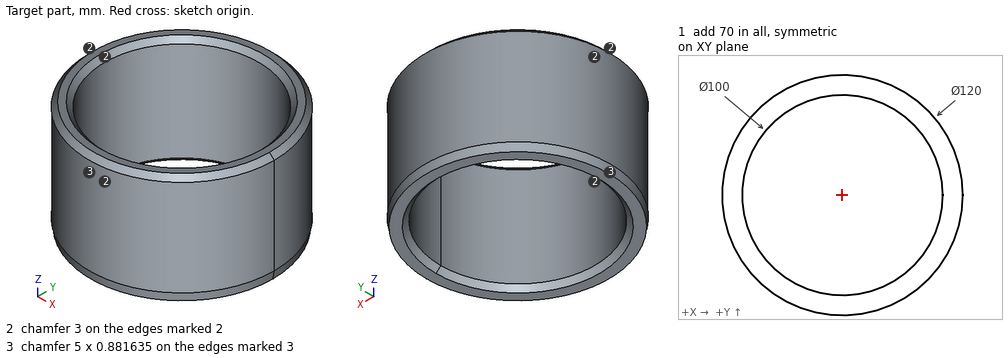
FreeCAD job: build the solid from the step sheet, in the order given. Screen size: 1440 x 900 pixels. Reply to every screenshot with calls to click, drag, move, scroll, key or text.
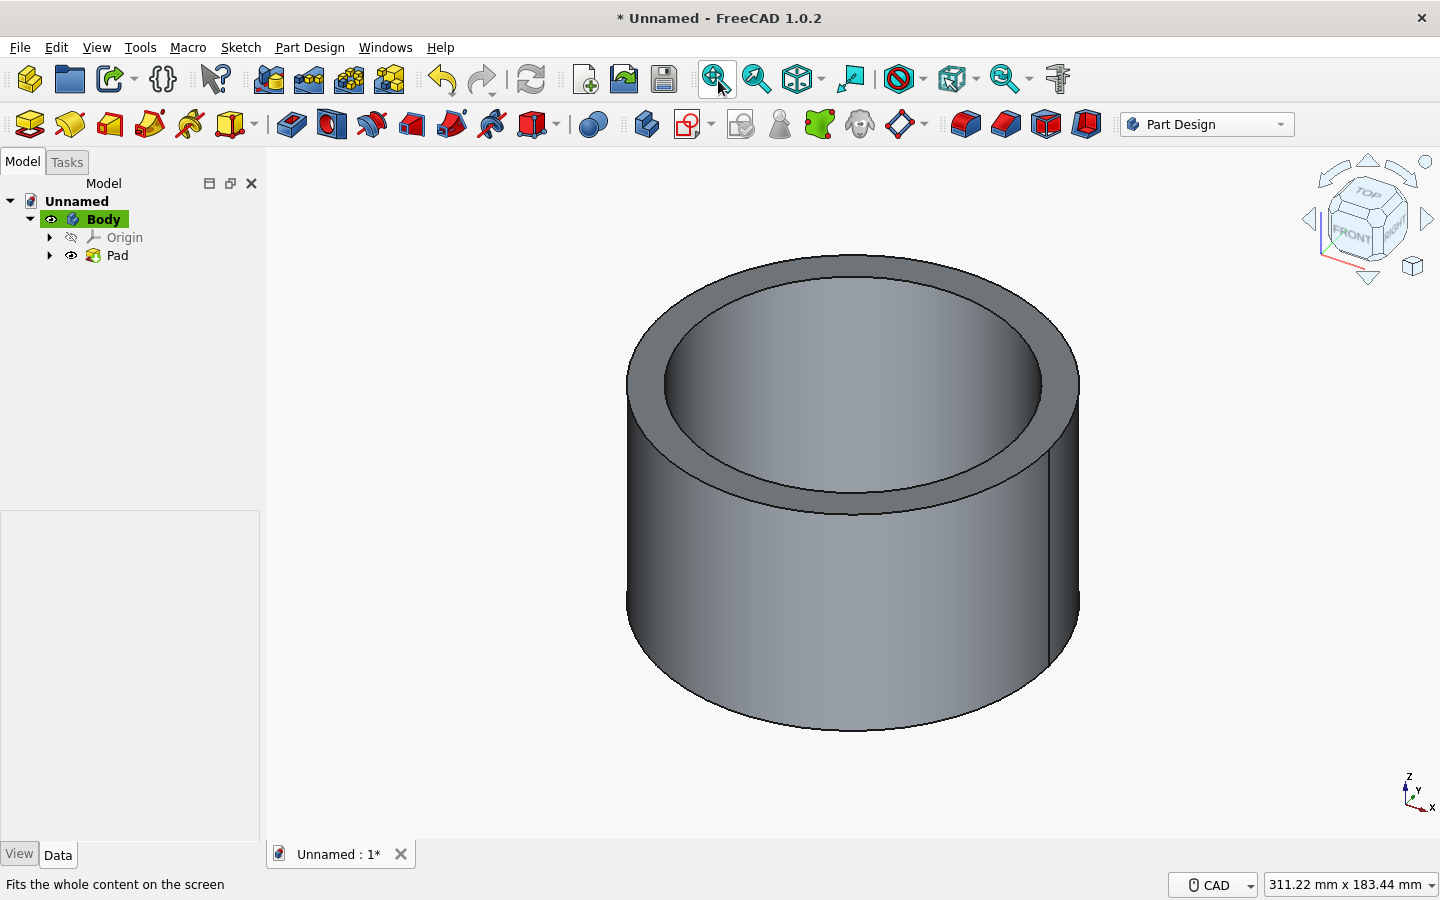
click(628, 397)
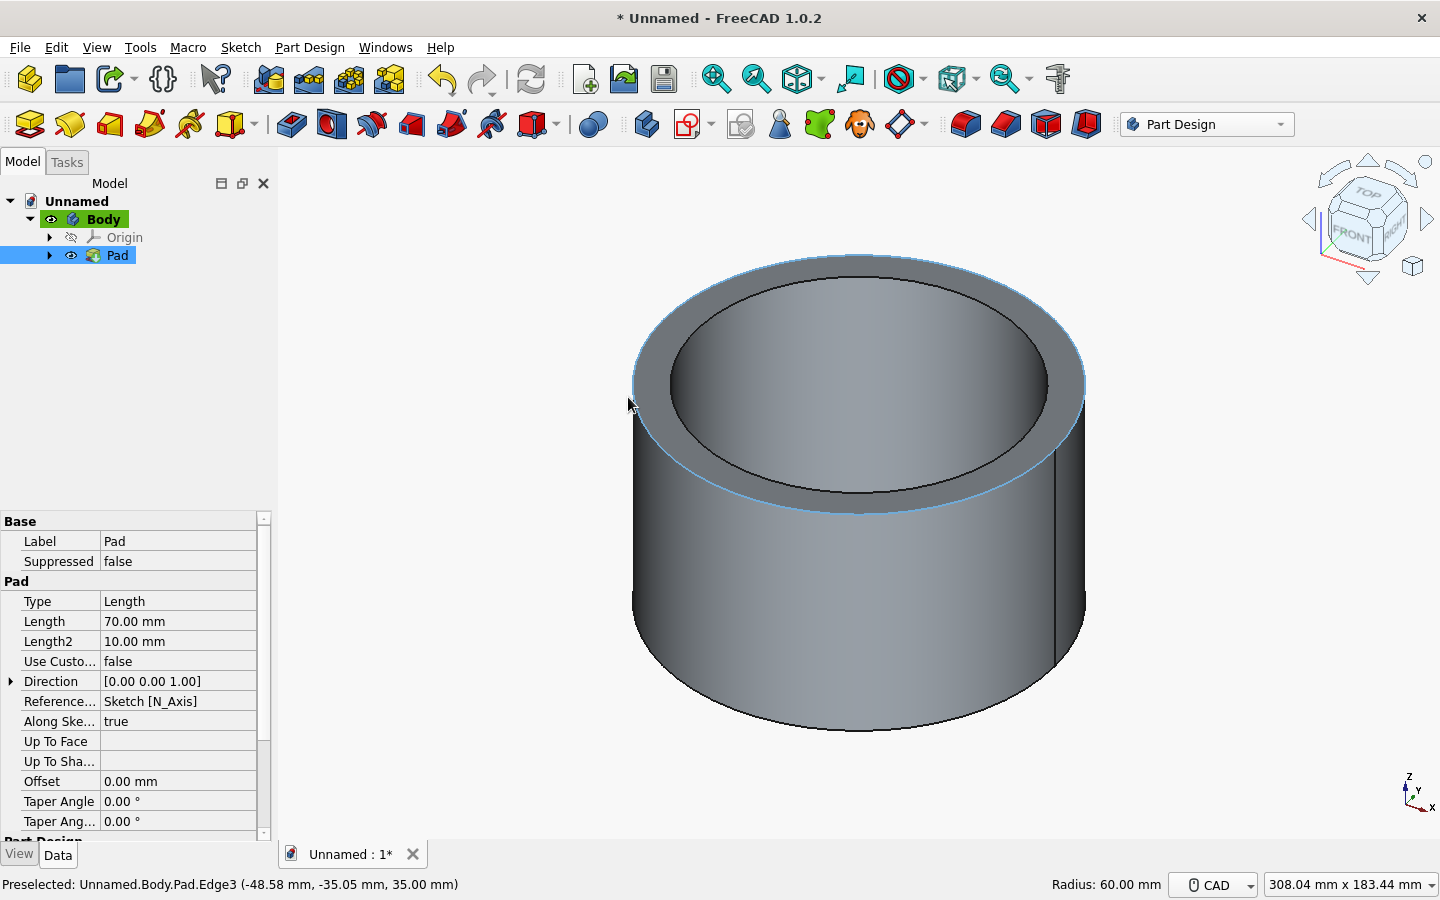
click(696, 330, ctrl)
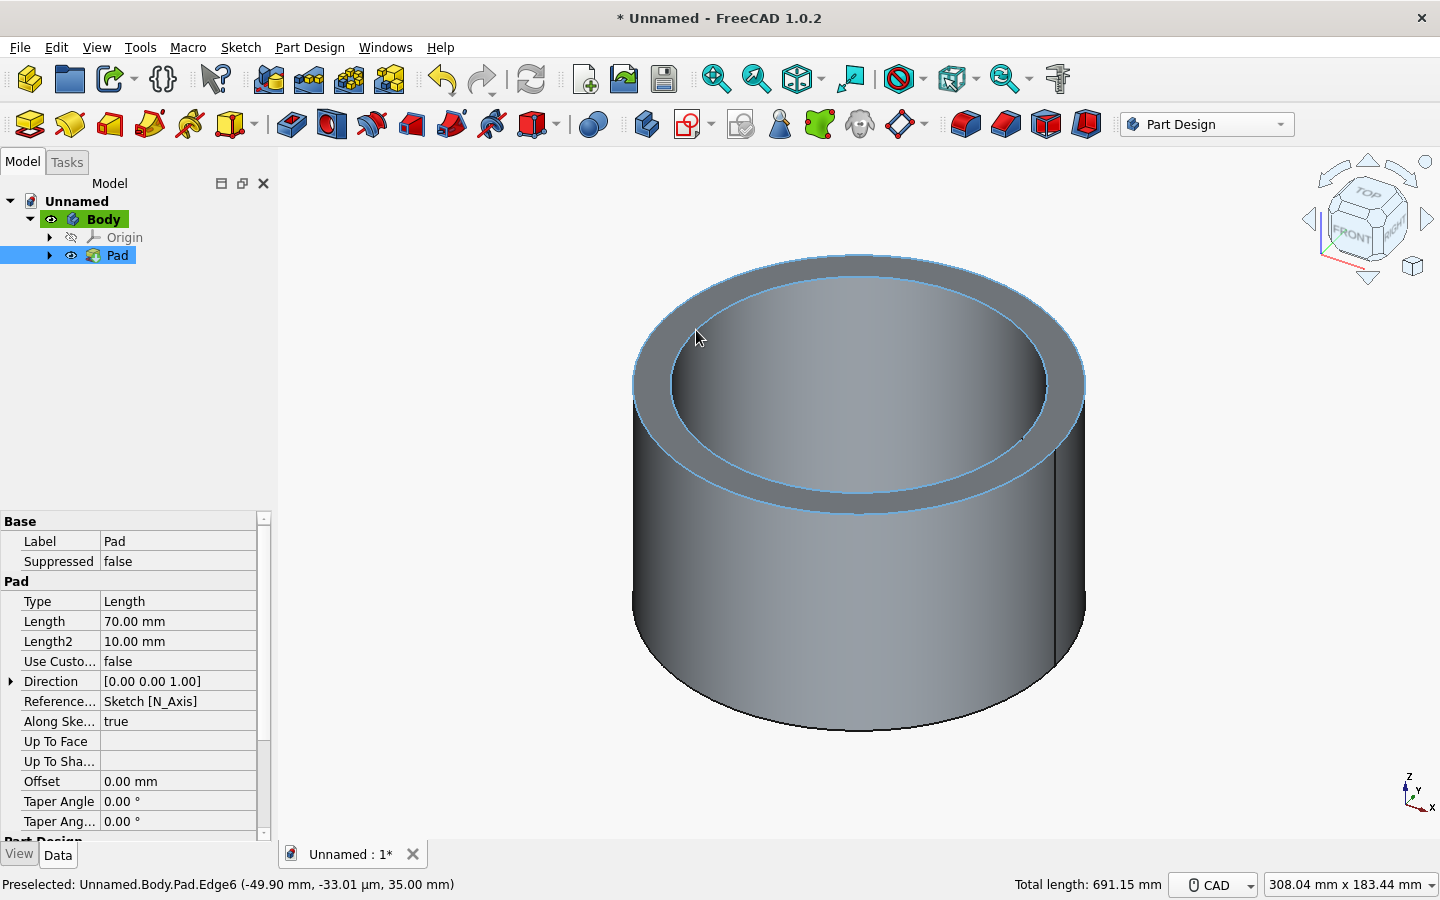
key(0)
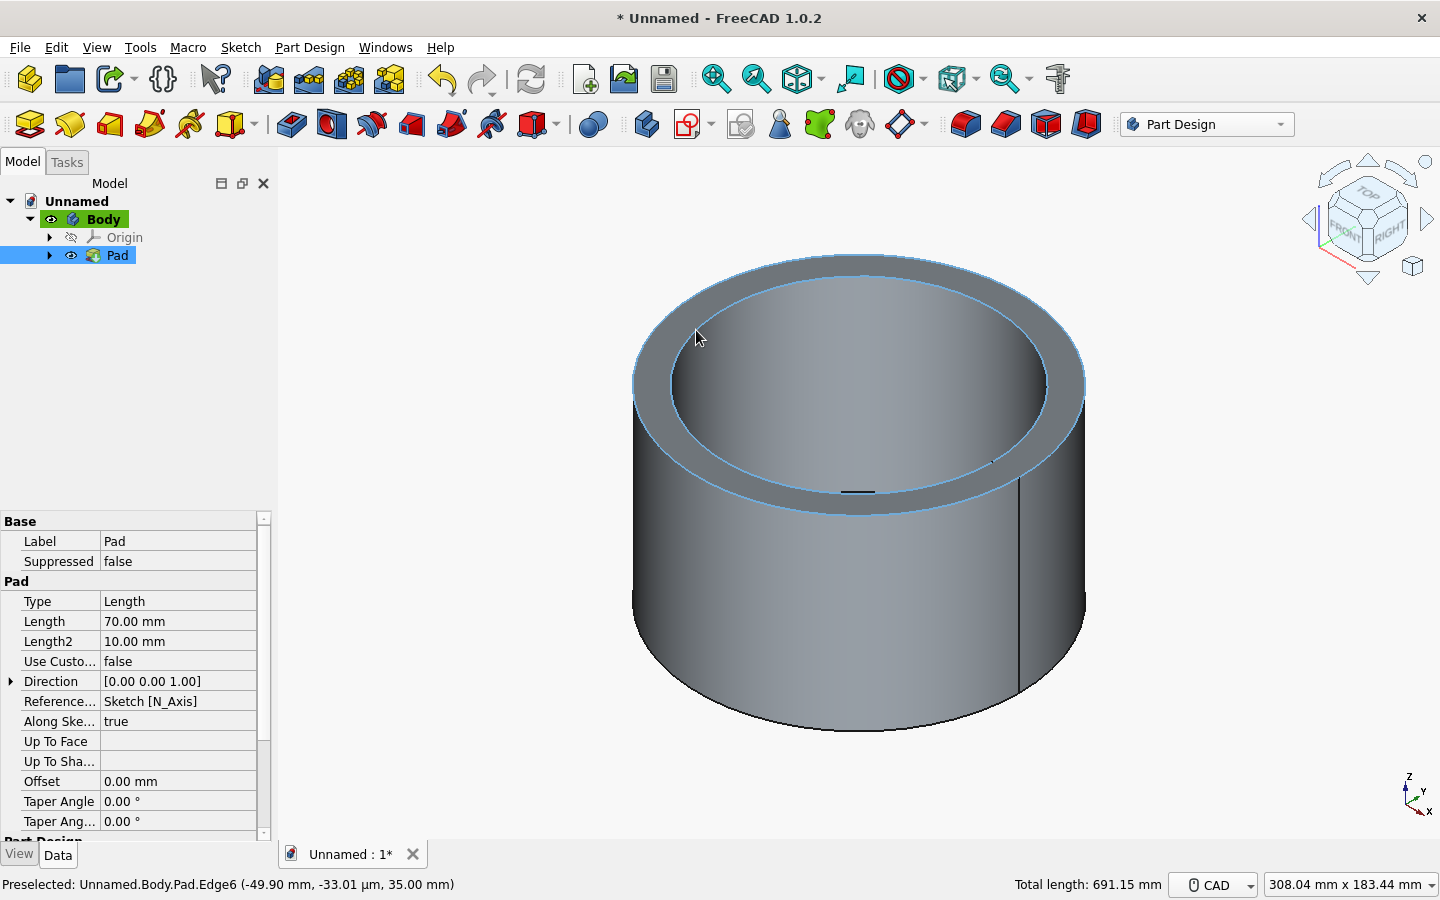
key(2)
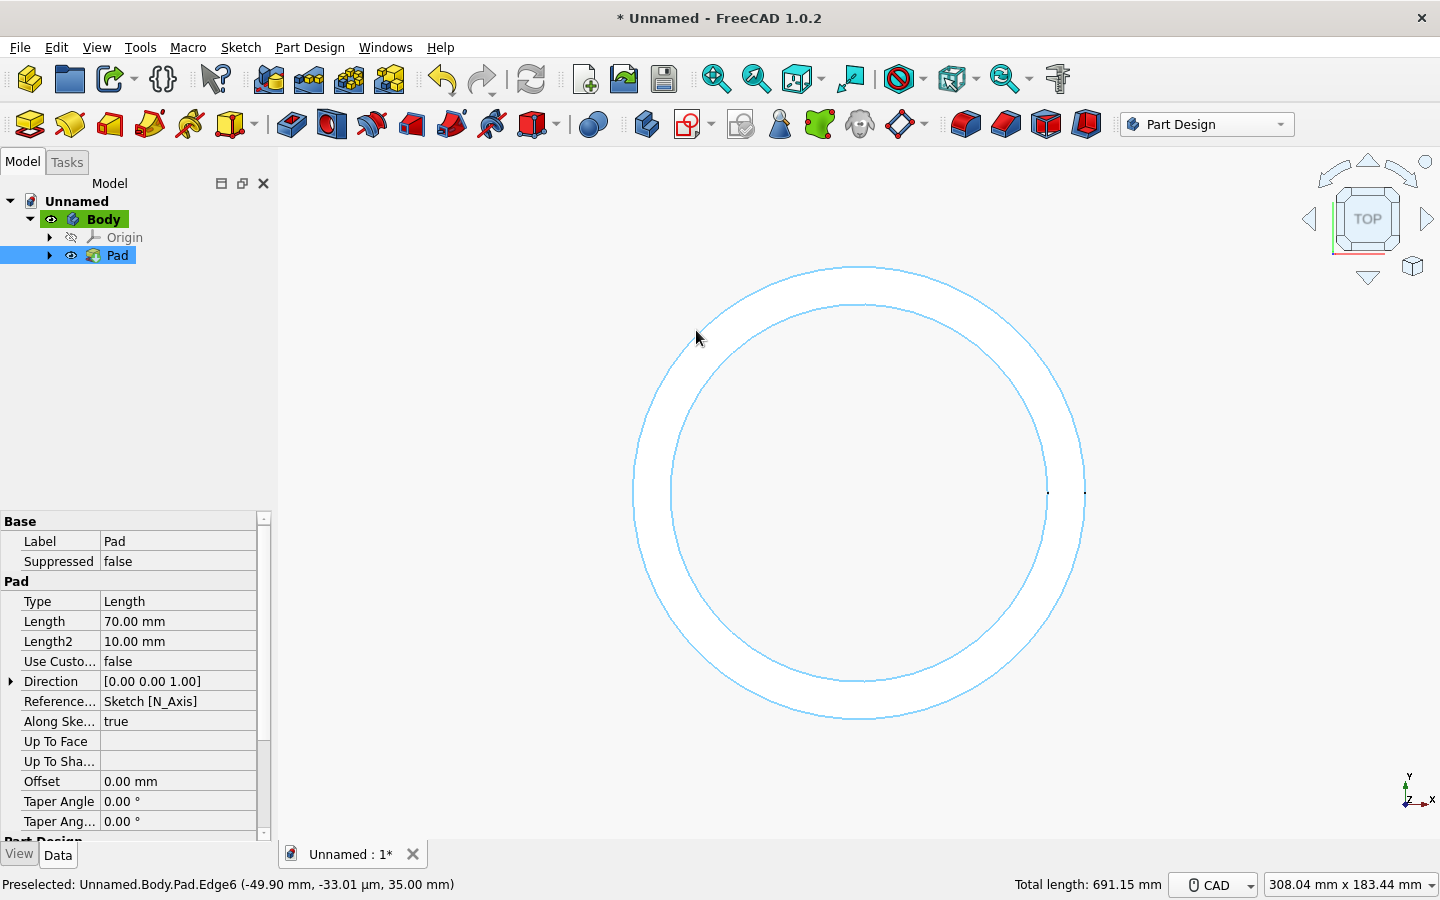
key(1)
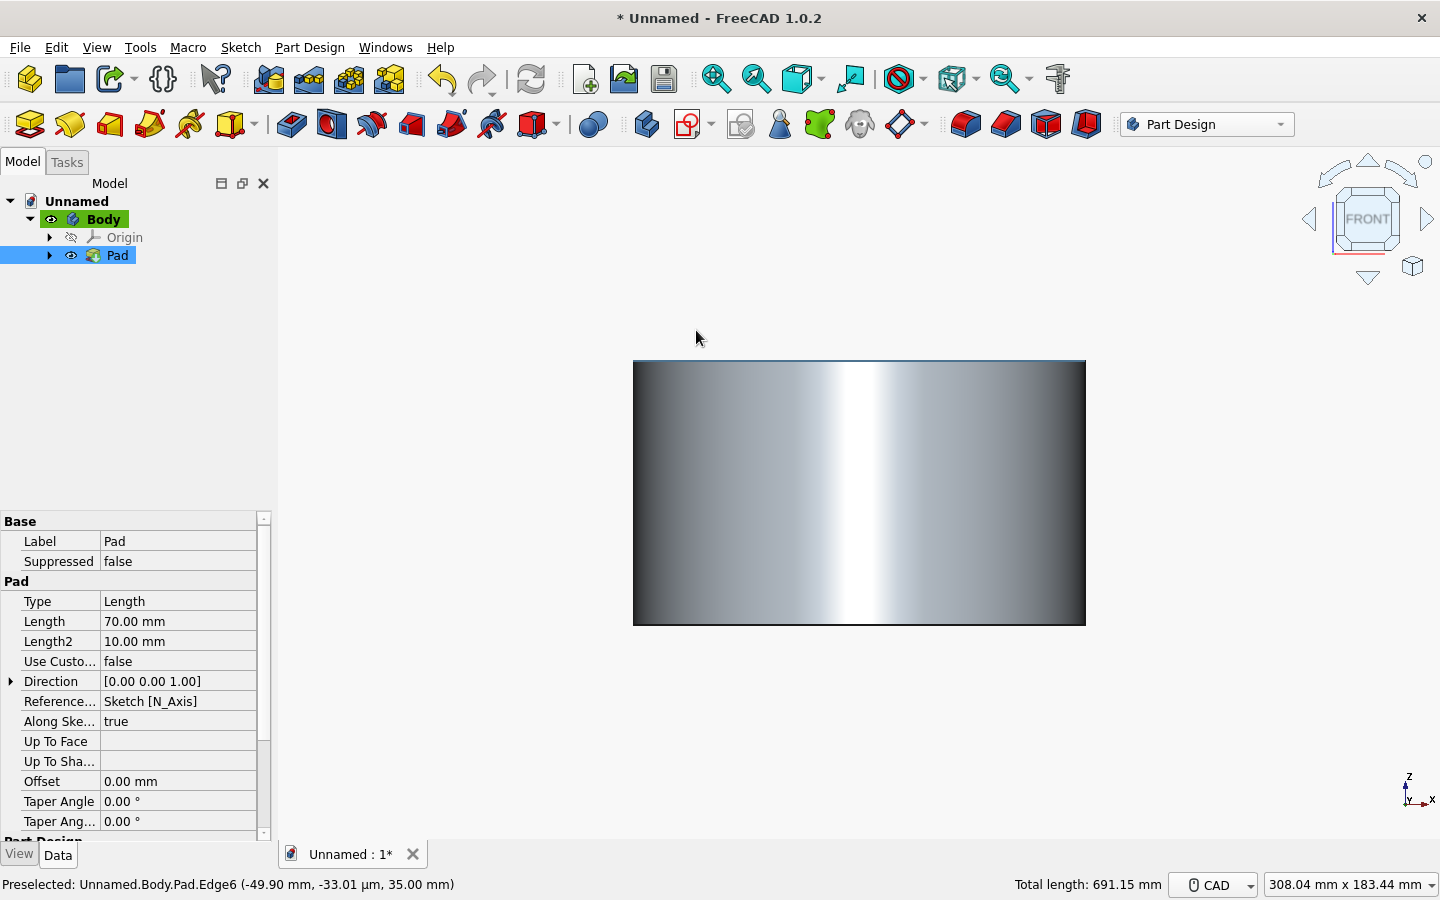
click(718, 80)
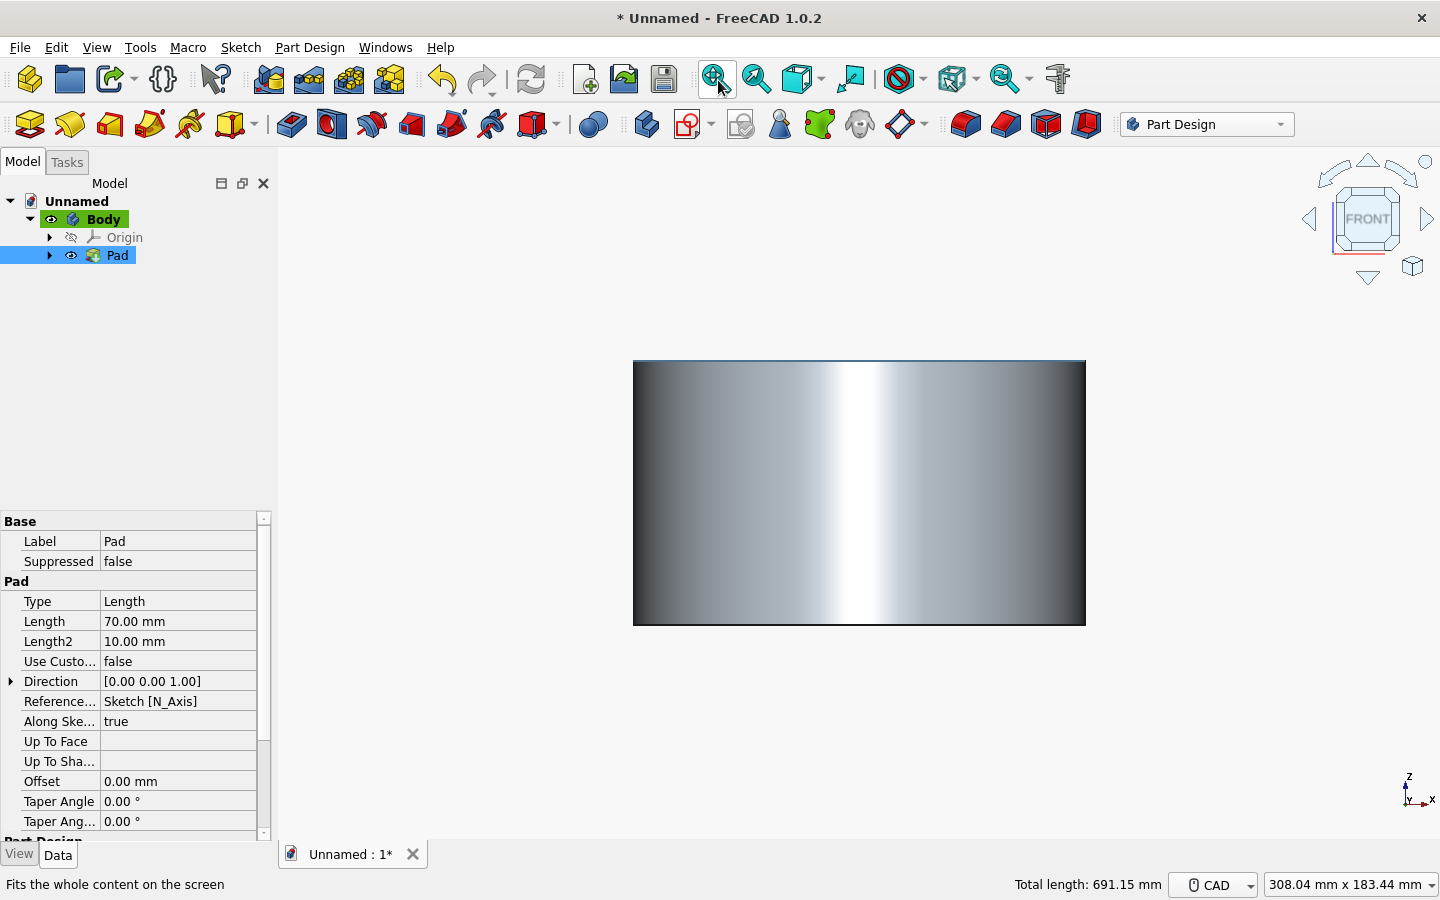
key(3)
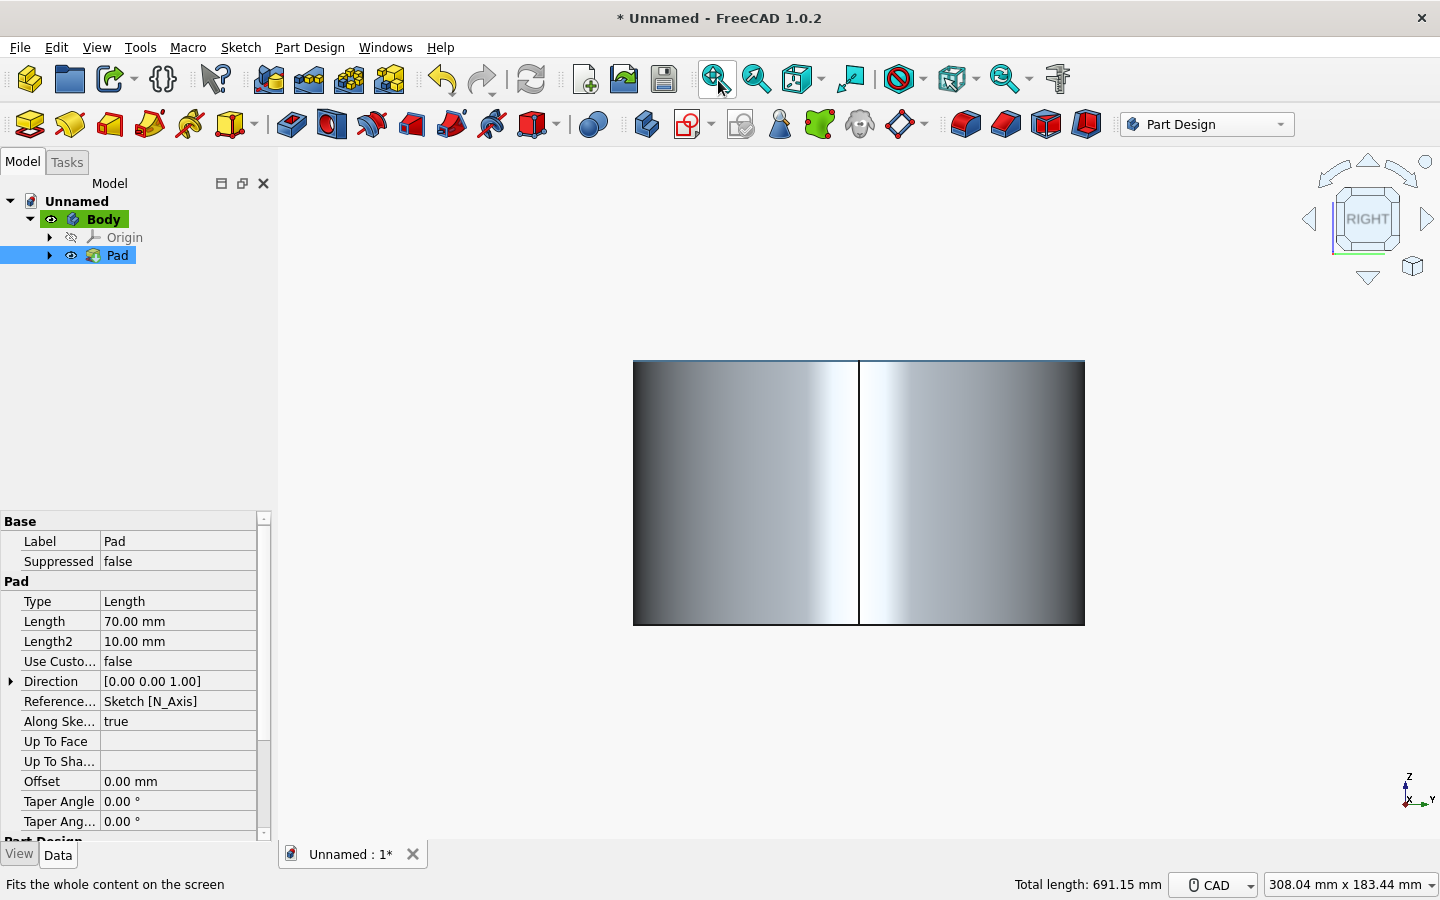
click(718, 80)